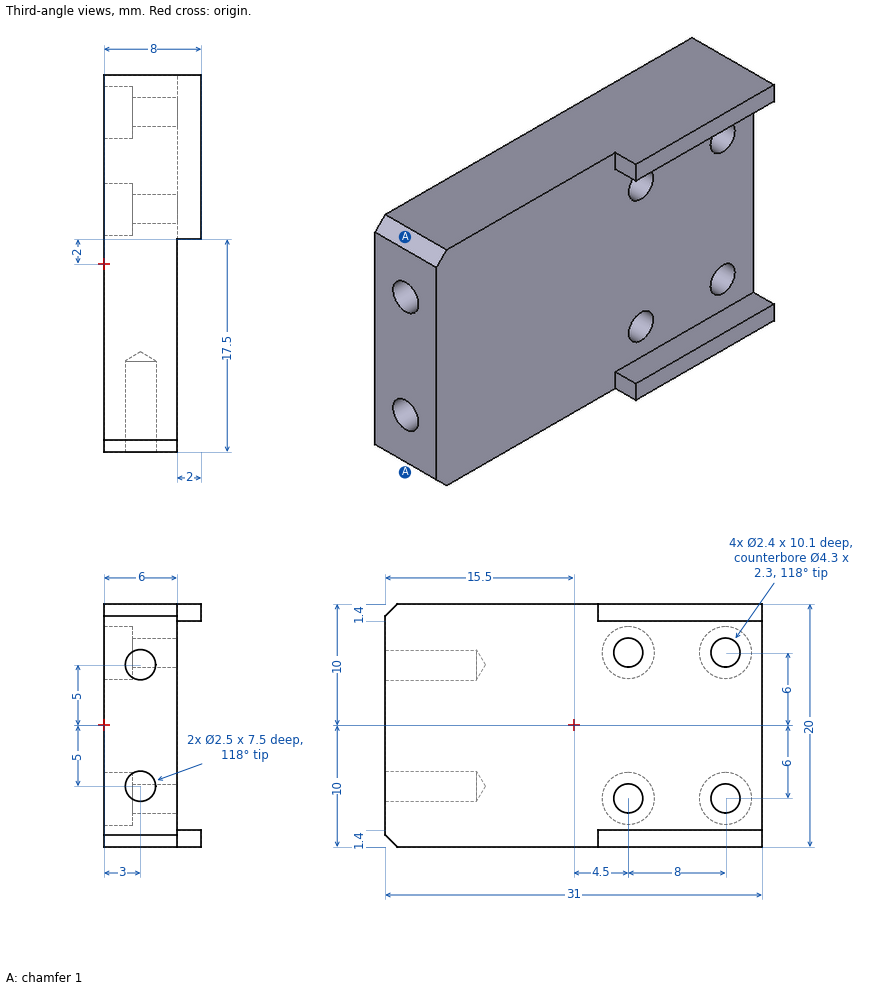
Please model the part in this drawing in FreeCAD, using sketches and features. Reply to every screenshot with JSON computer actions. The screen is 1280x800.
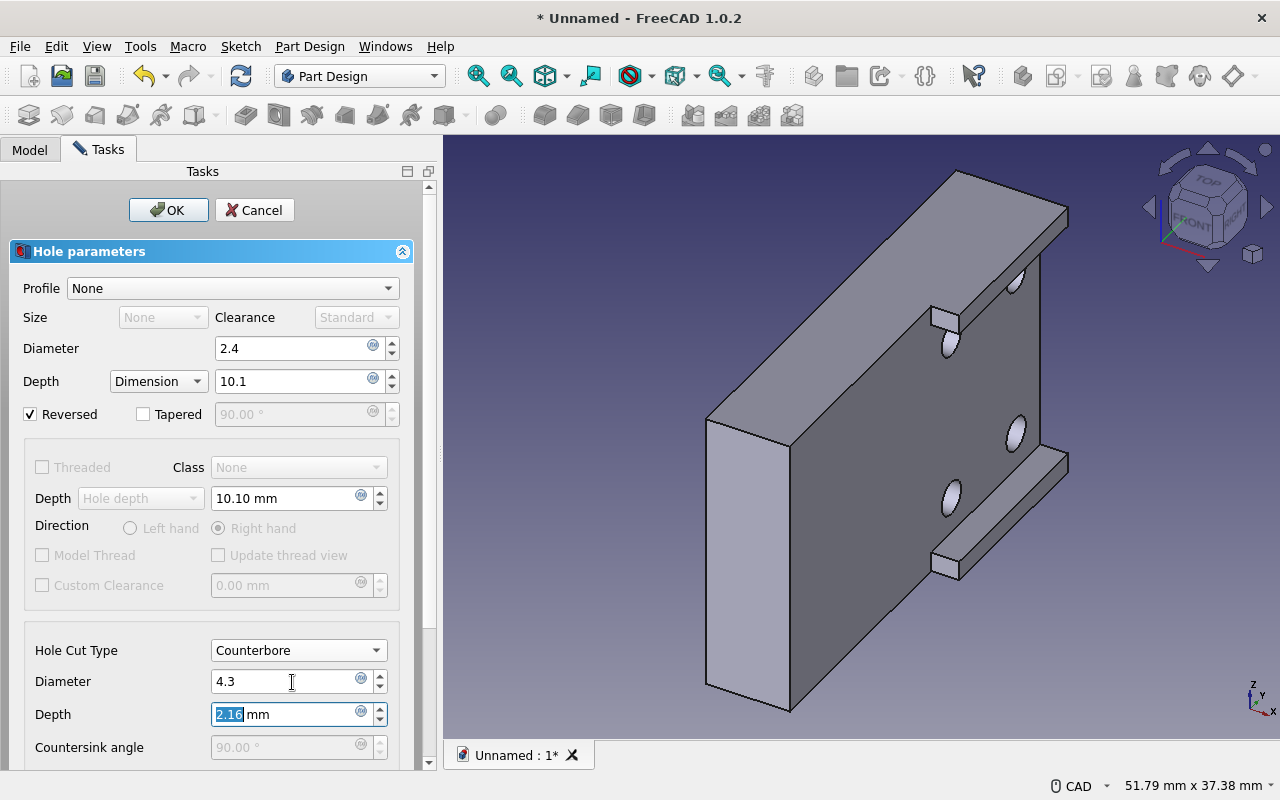
{"action": "type", "text": "2.3"}
{"action": "key", "text": "Tab"}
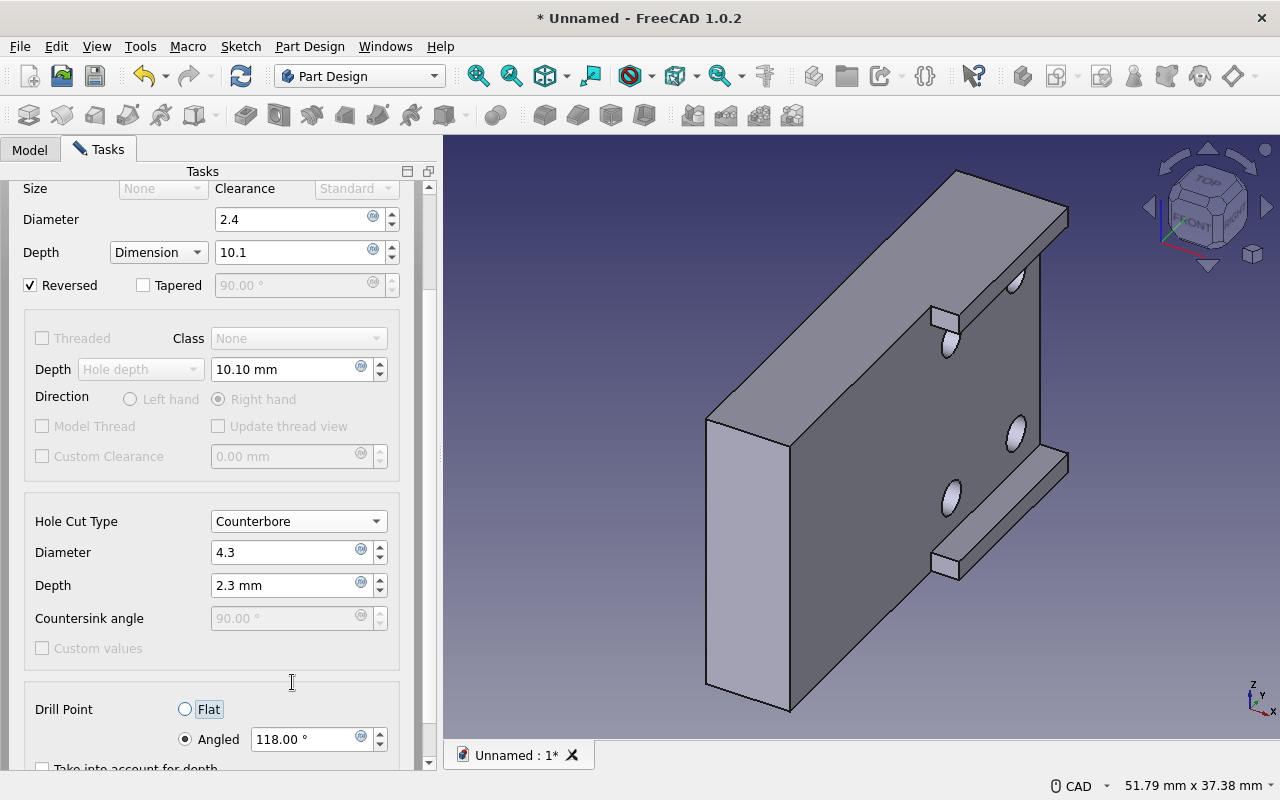
{"action": "scroll", "coordinate": [429, 476], "scroll_direction": "up", "scroll_amount": 3}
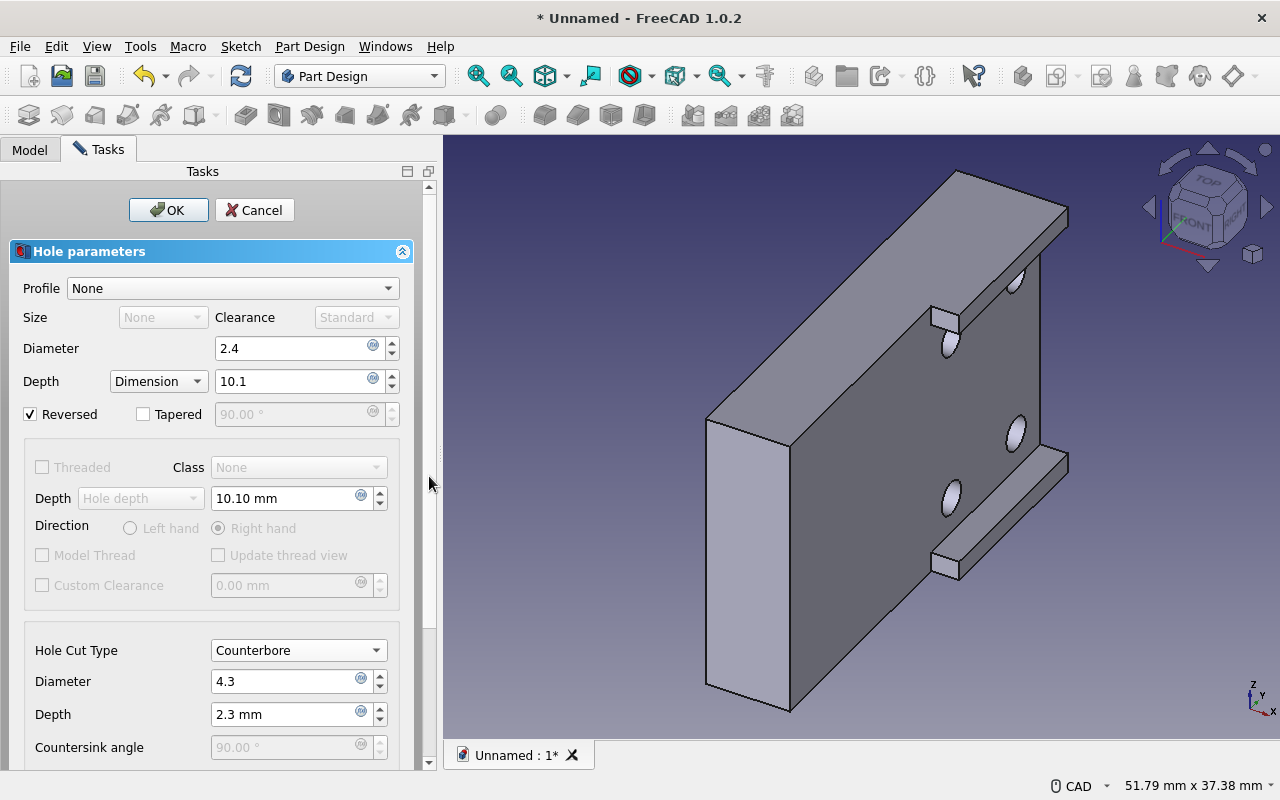
{"action": "left_click", "coordinate": [169, 210]}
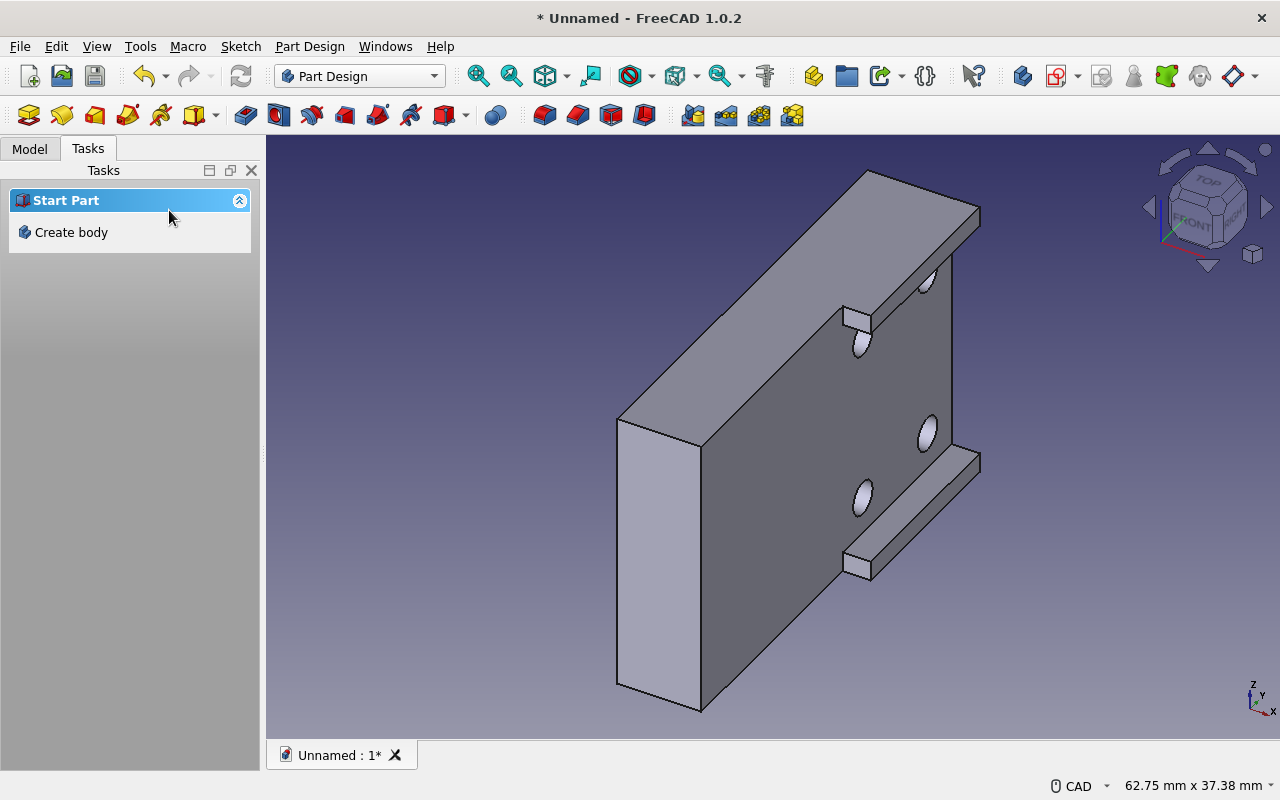
{"action": "left_click", "coordinate": [659, 489]}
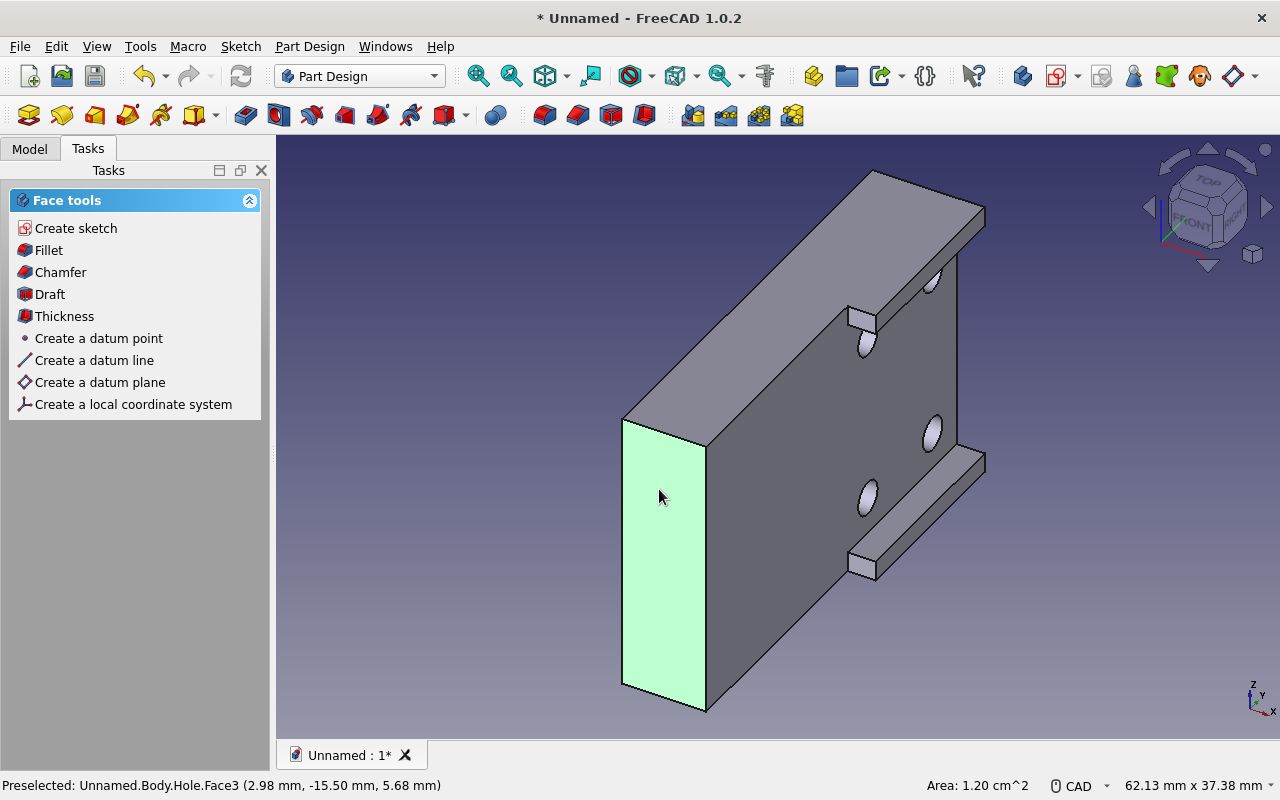
{"action": "left_click", "coordinate": [1056, 76]}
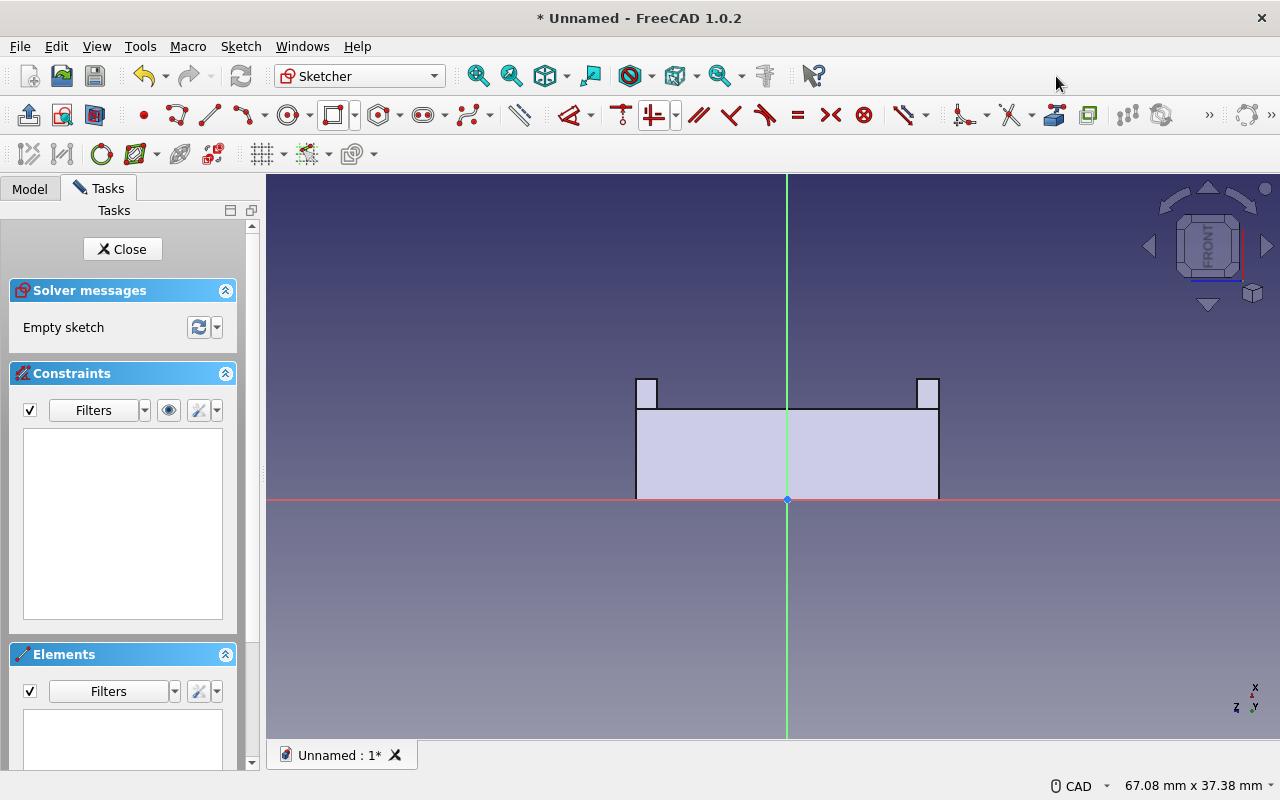
{"action": "scroll", "coordinate": [823, 472], "scroll_direction": "up", "scroll_amount": 6}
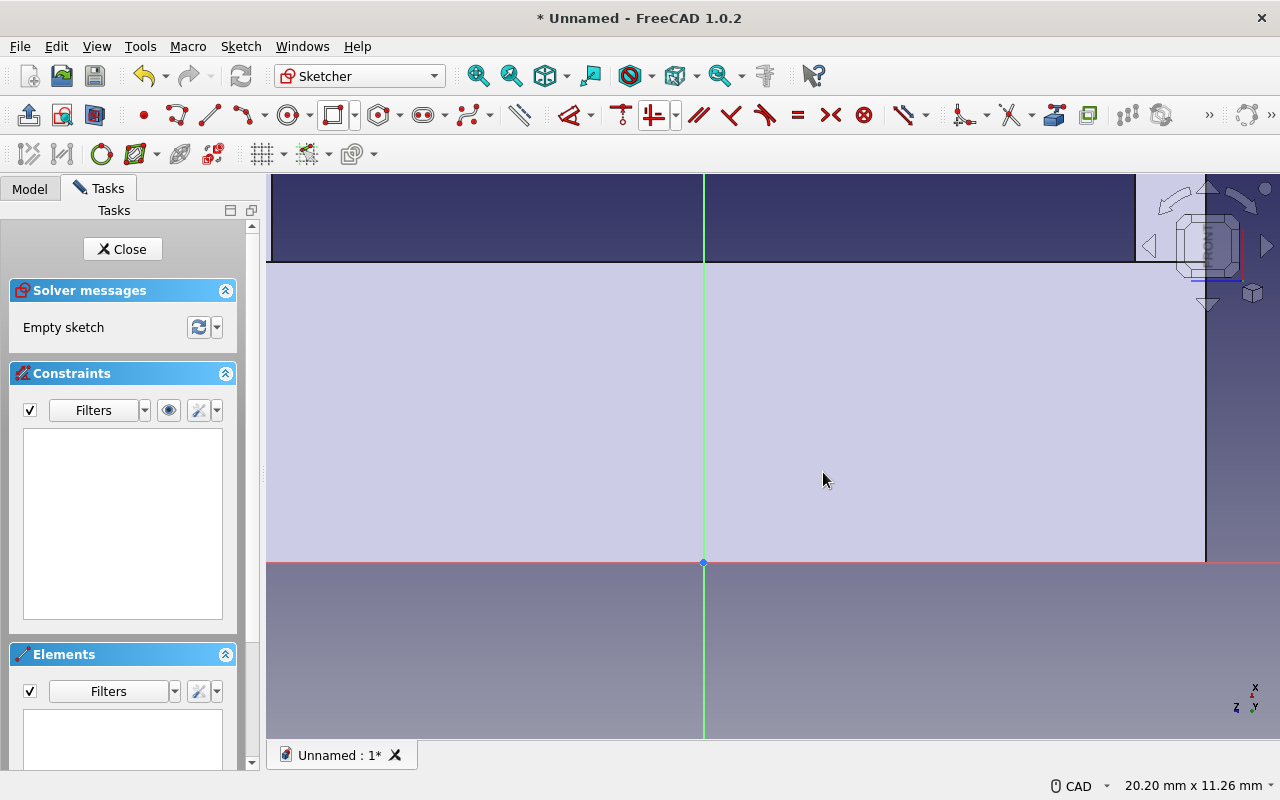
{"action": "left_click", "coordinate": [288, 116]}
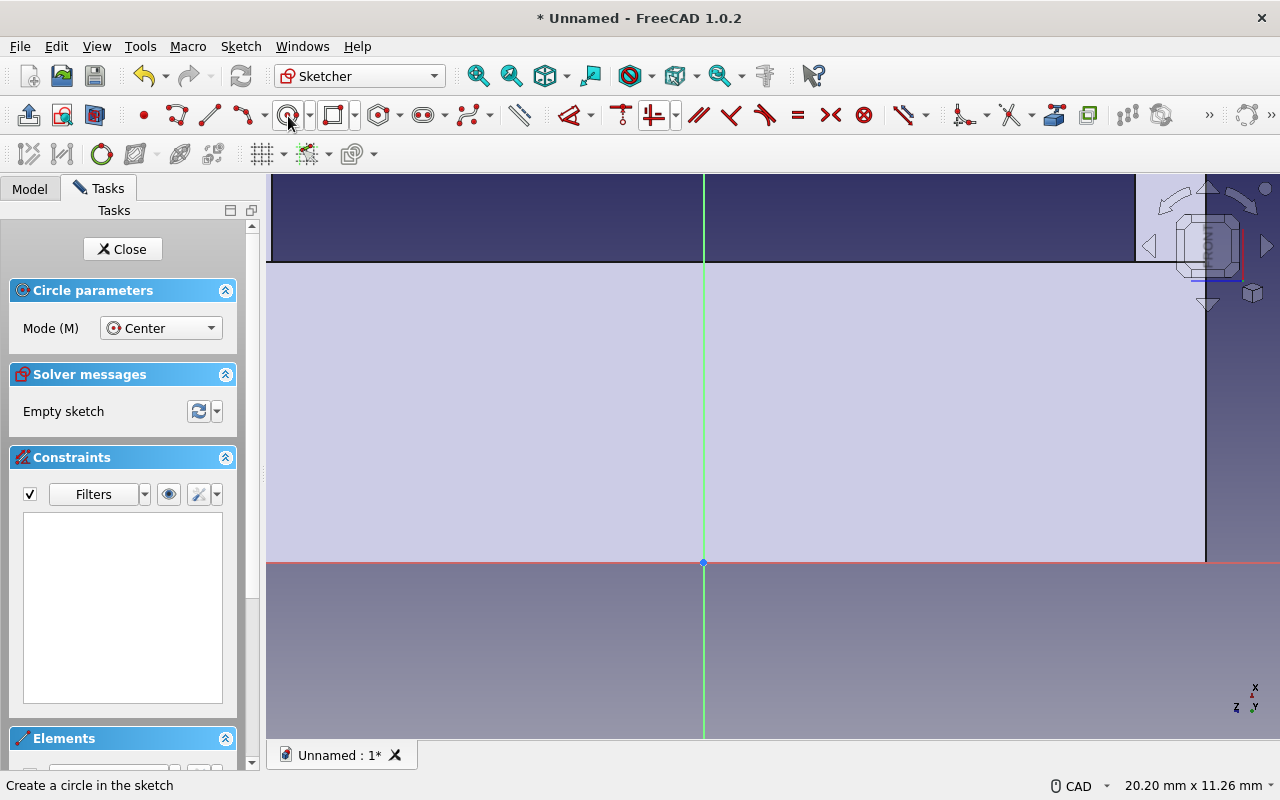
{"action": "left_click", "coordinate": [955, 412]}
{"action": "left_click", "coordinate": [999, 368]}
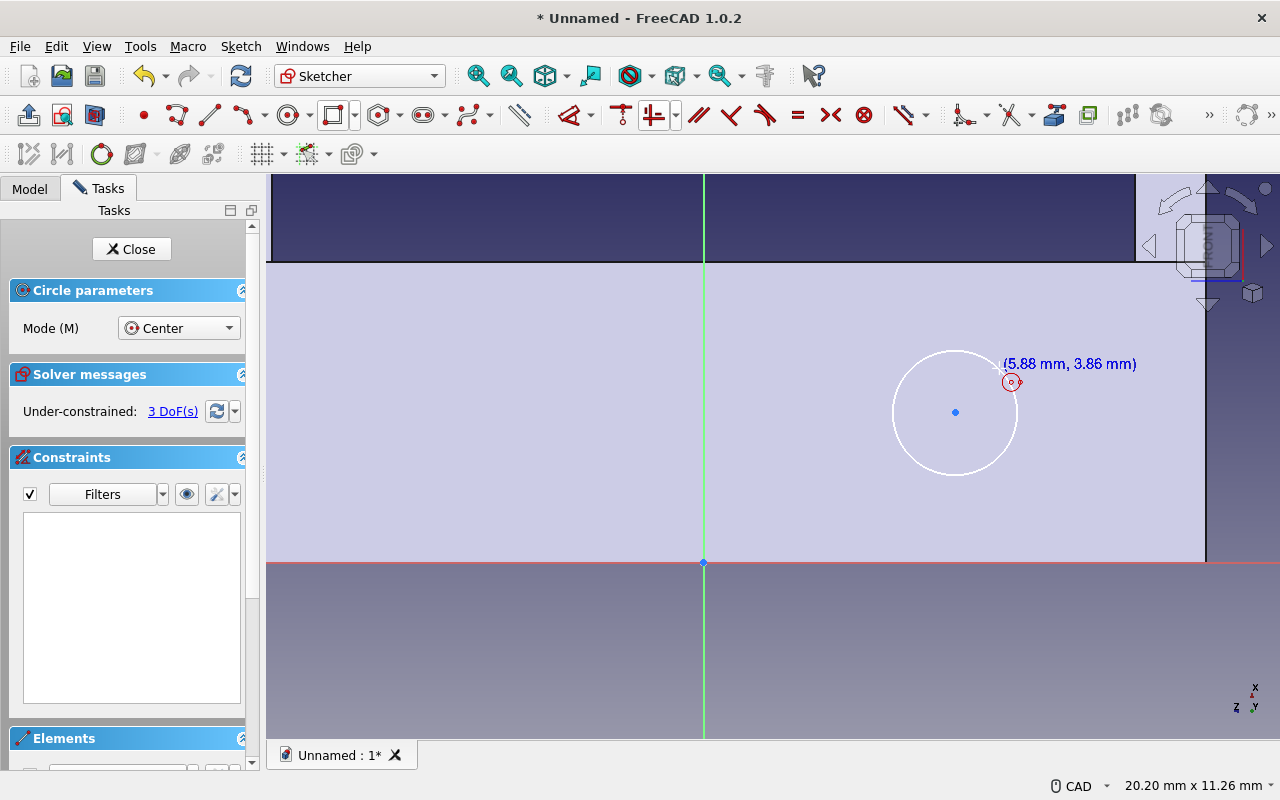
{"action": "left_click", "coordinate": [453, 412]}
{"action": "left_click", "coordinate": [497, 368]}
{"action": "key", "text": "Escape"}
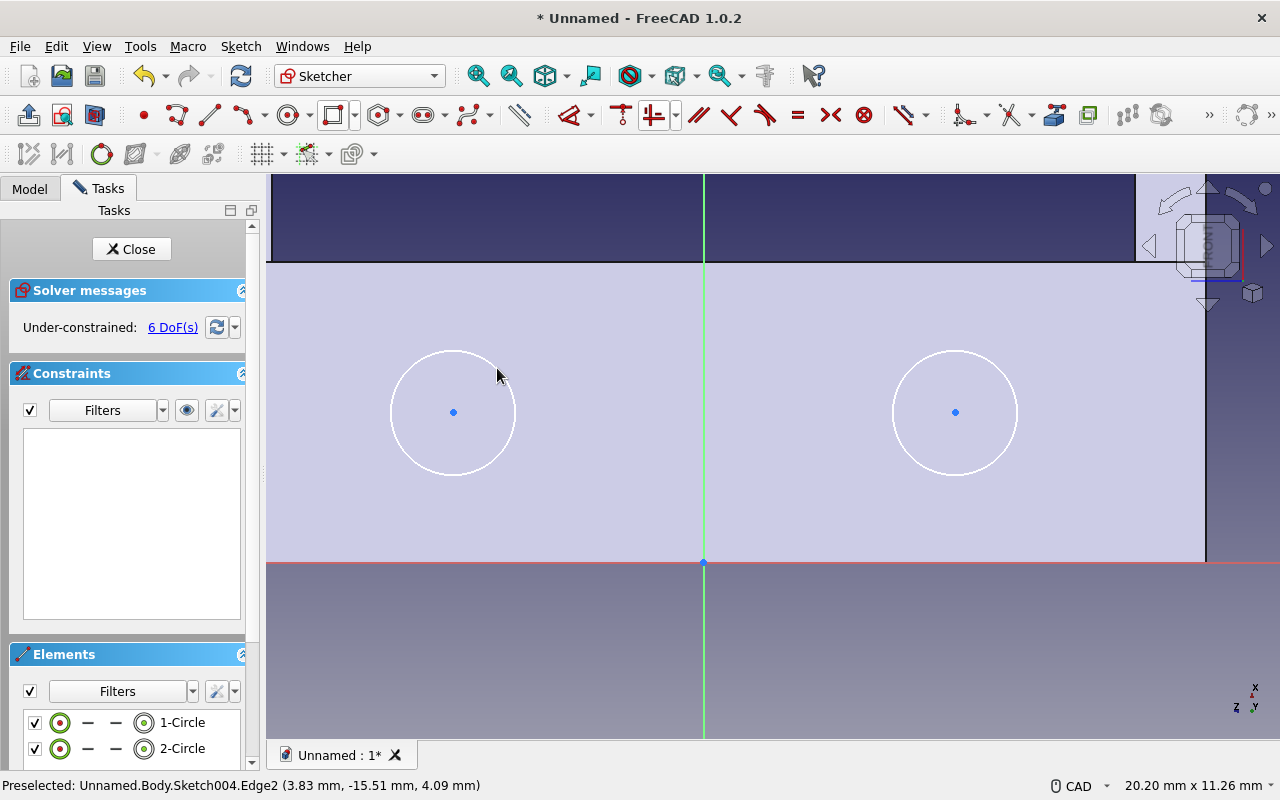
{"action": "left_click", "coordinate": [999, 369]}